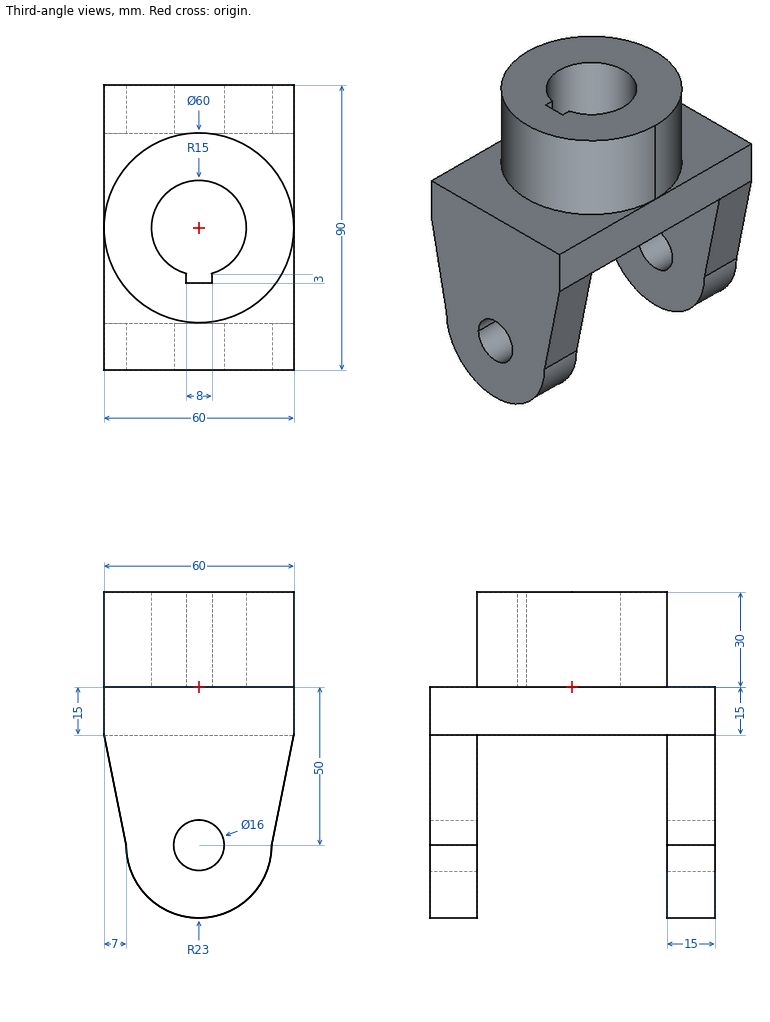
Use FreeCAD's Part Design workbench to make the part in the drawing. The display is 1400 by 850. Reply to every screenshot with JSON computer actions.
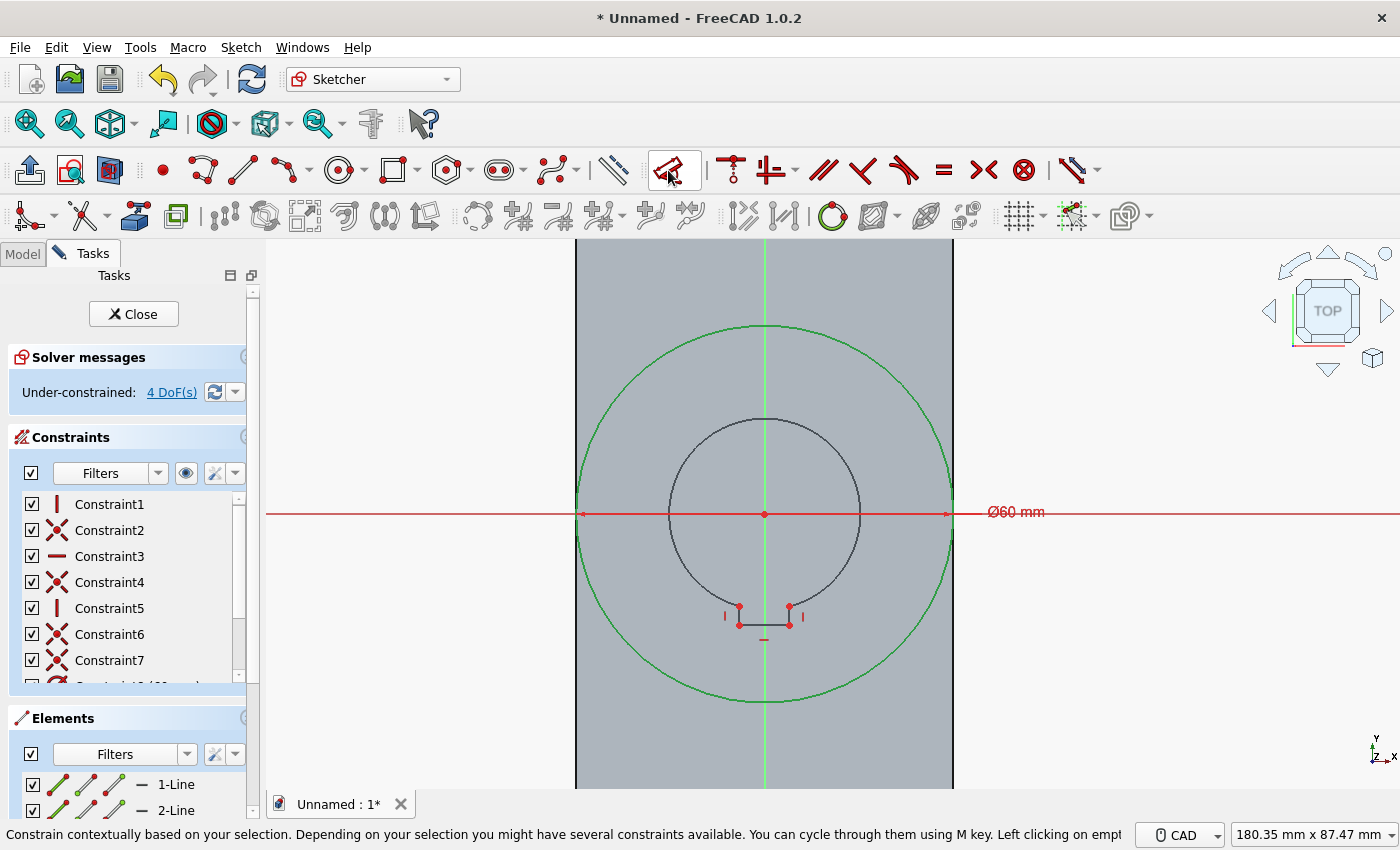
{"action": "left_click", "coordinate": [852, 476]}
{"action": "left_click", "coordinate": [881, 463]}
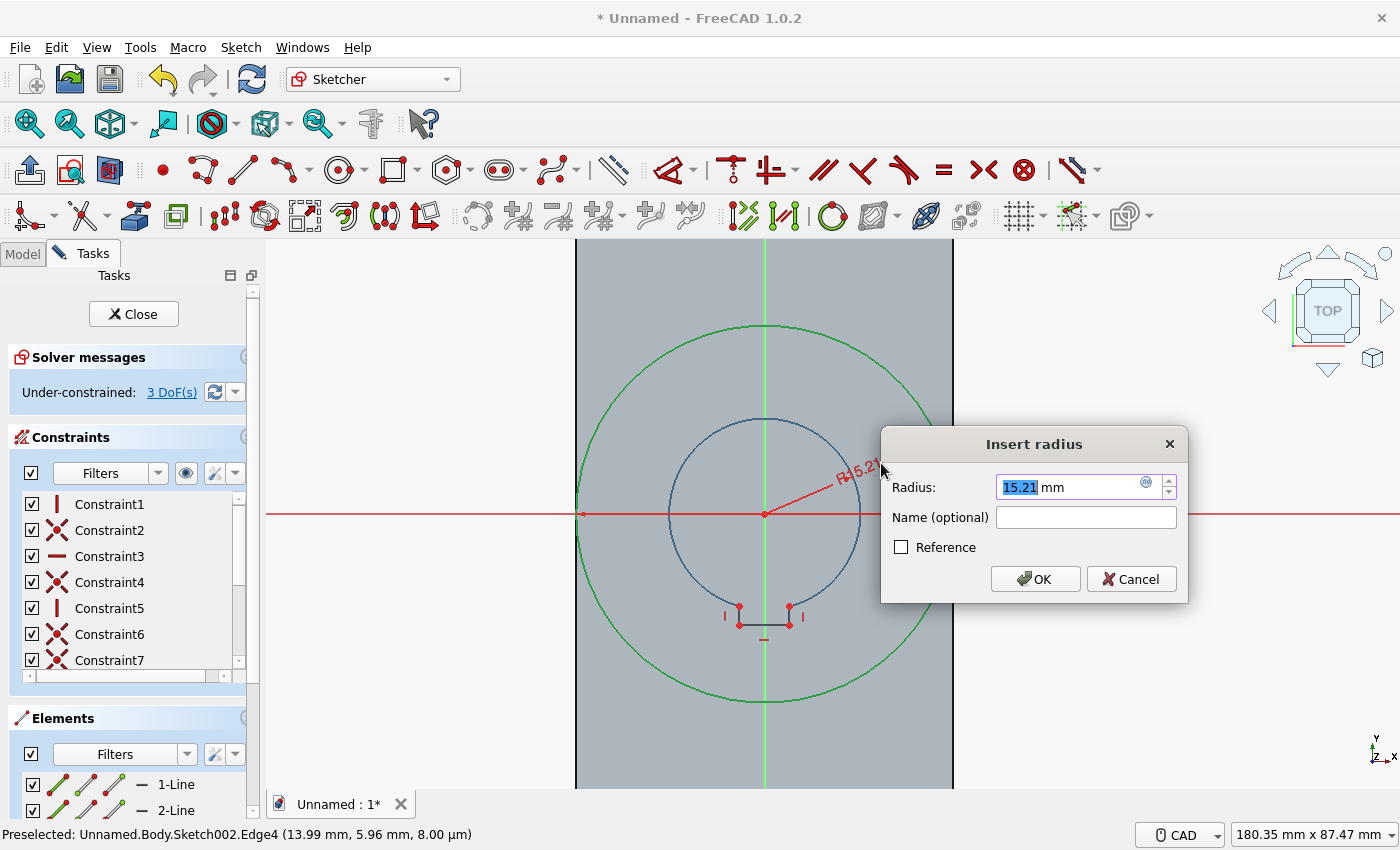
{"action": "type", "text": "15"}
{"action": "key", "text": "Return"}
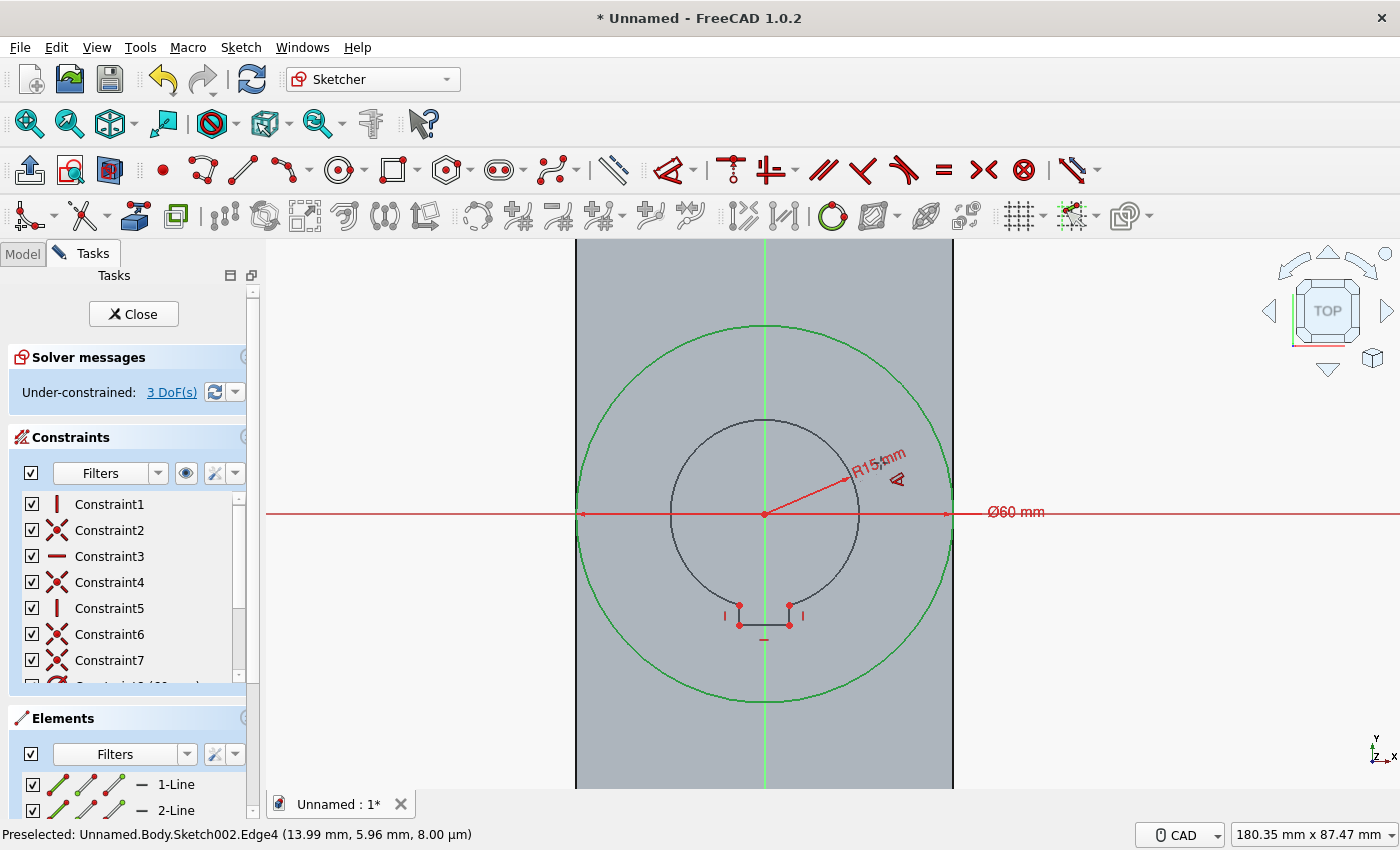
{"action": "scroll", "coordinate": [789, 615], "scroll_direction": "up", "scroll_amount": 4}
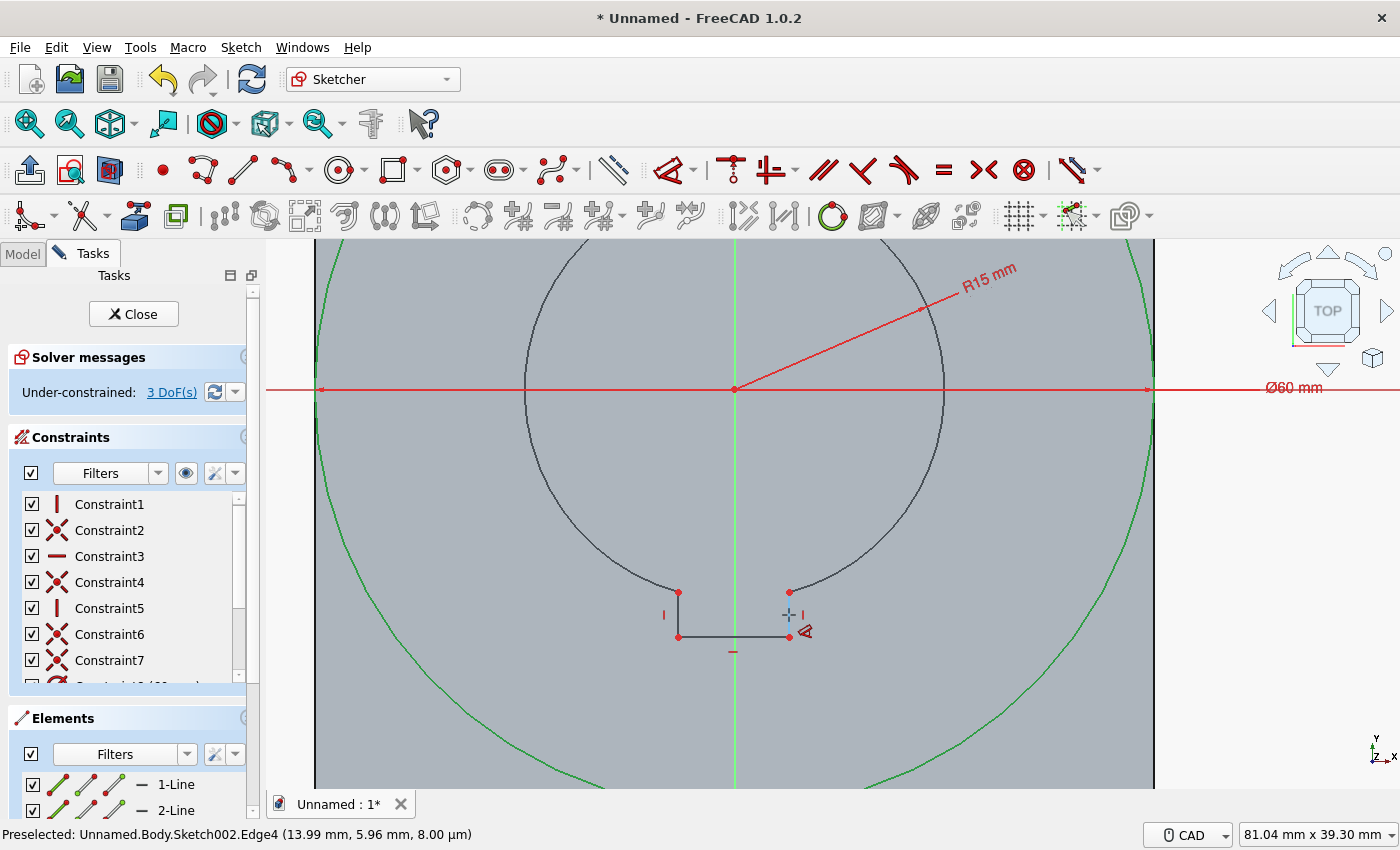
{"action": "left_click", "coordinate": [789, 615]}
{"action": "left_click", "coordinate": [823, 615]}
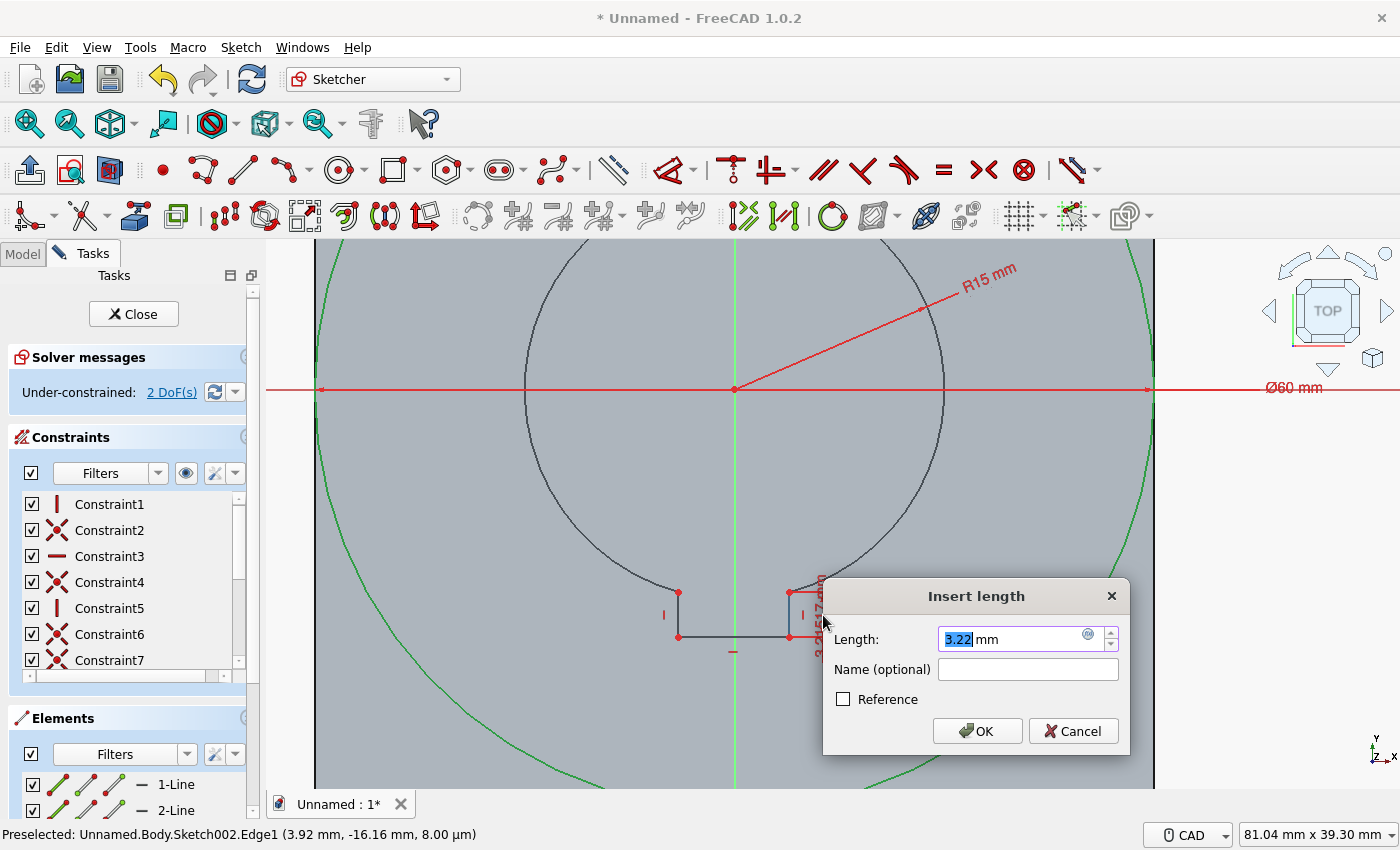
{"action": "type", "text": "3"}
{"action": "key", "text": "Return"}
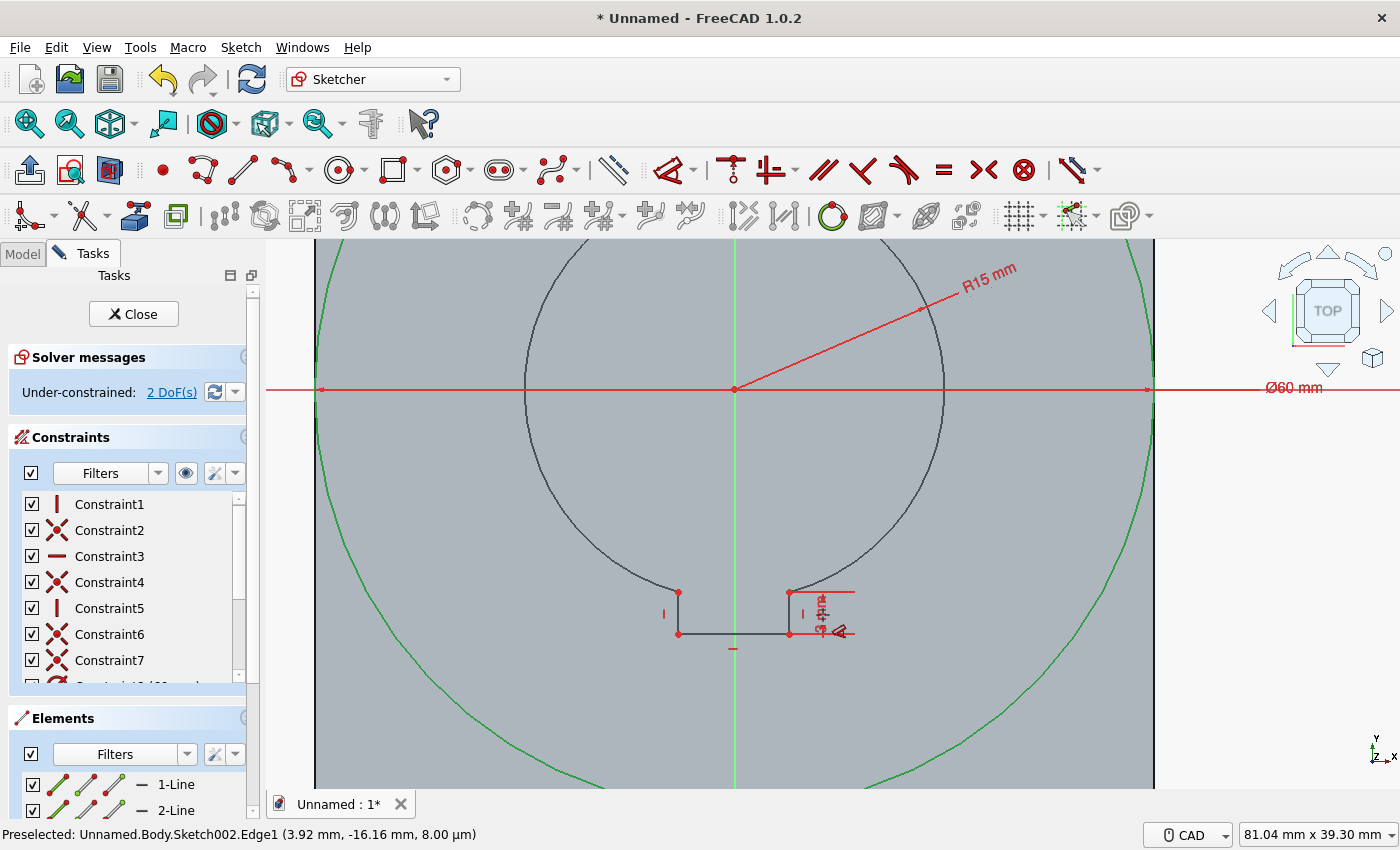
{"action": "left_click", "coordinate": [756, 634]}
{"action": "left_click", "coordinate": [708, 668]}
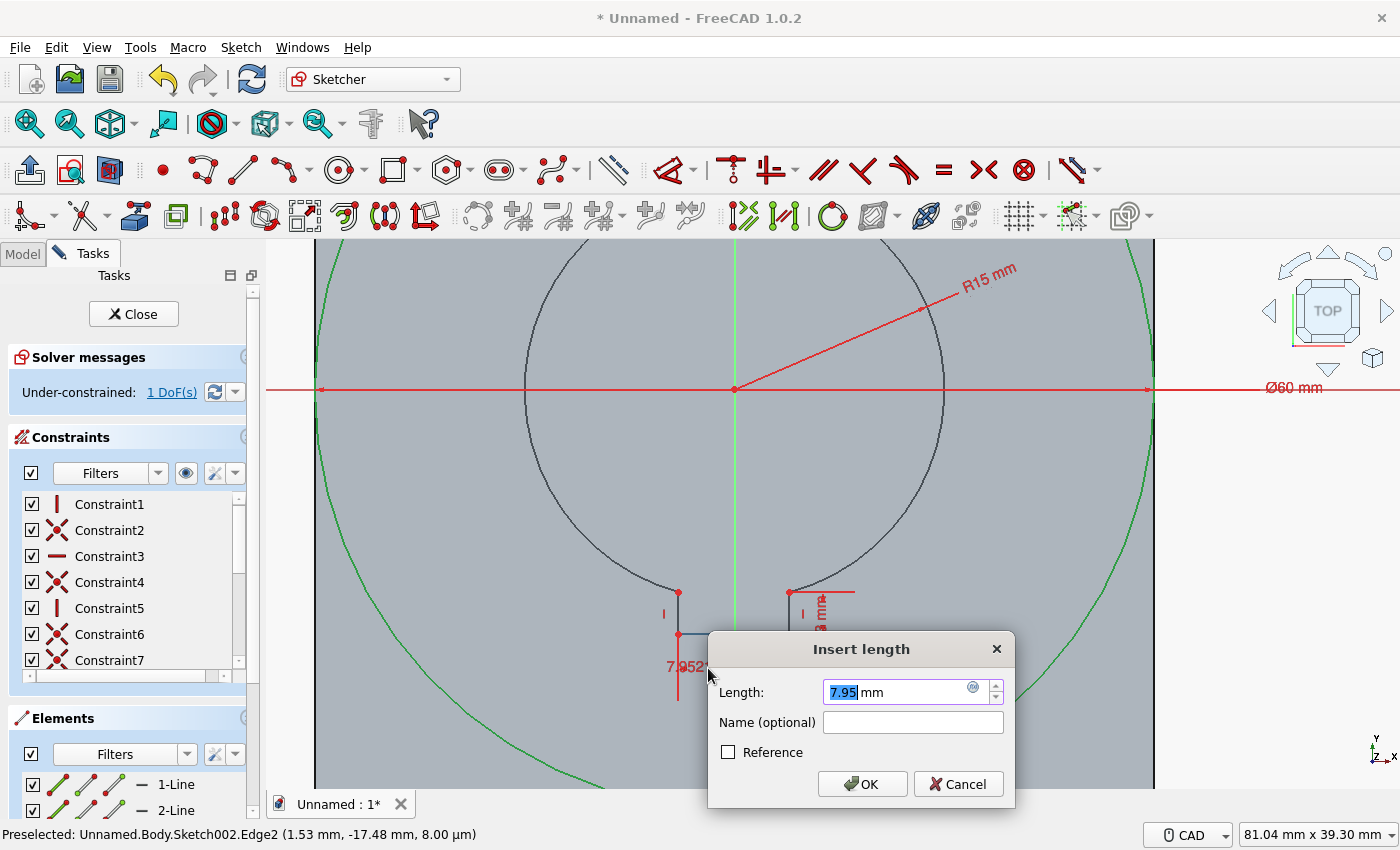
{"action": "type", "text": "8"}
{"action": "key", "text": "Return"}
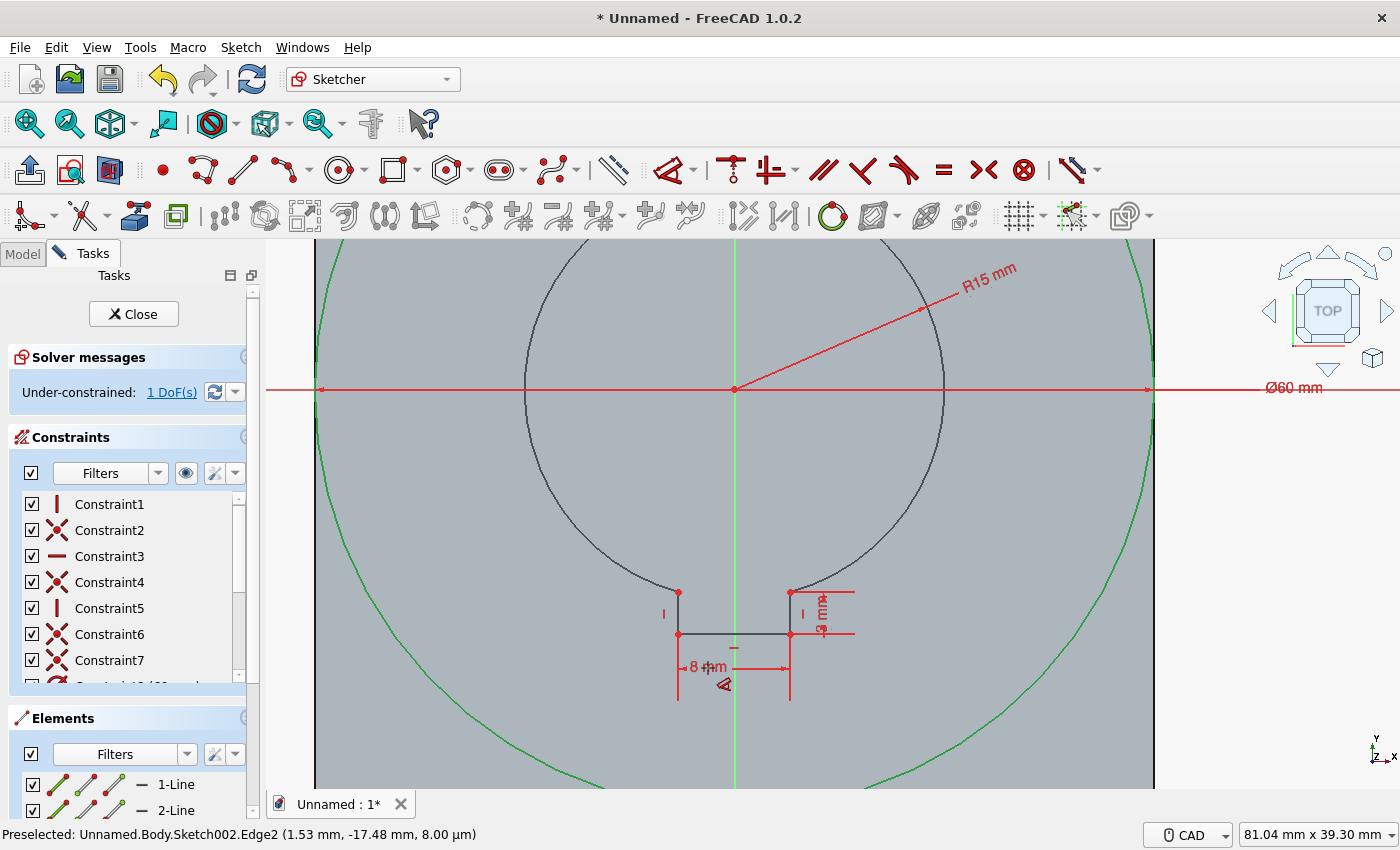
{"action": "left_click", "coordinate": [678, 622]}
{"action": "left_click", "coordinate": [644, 613]}